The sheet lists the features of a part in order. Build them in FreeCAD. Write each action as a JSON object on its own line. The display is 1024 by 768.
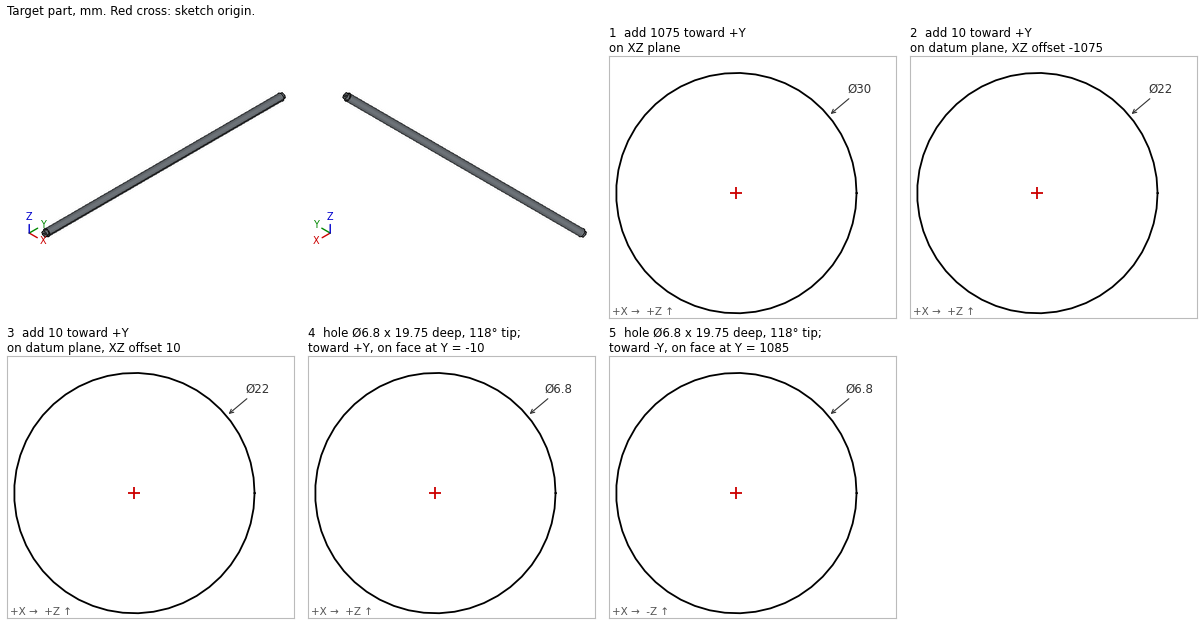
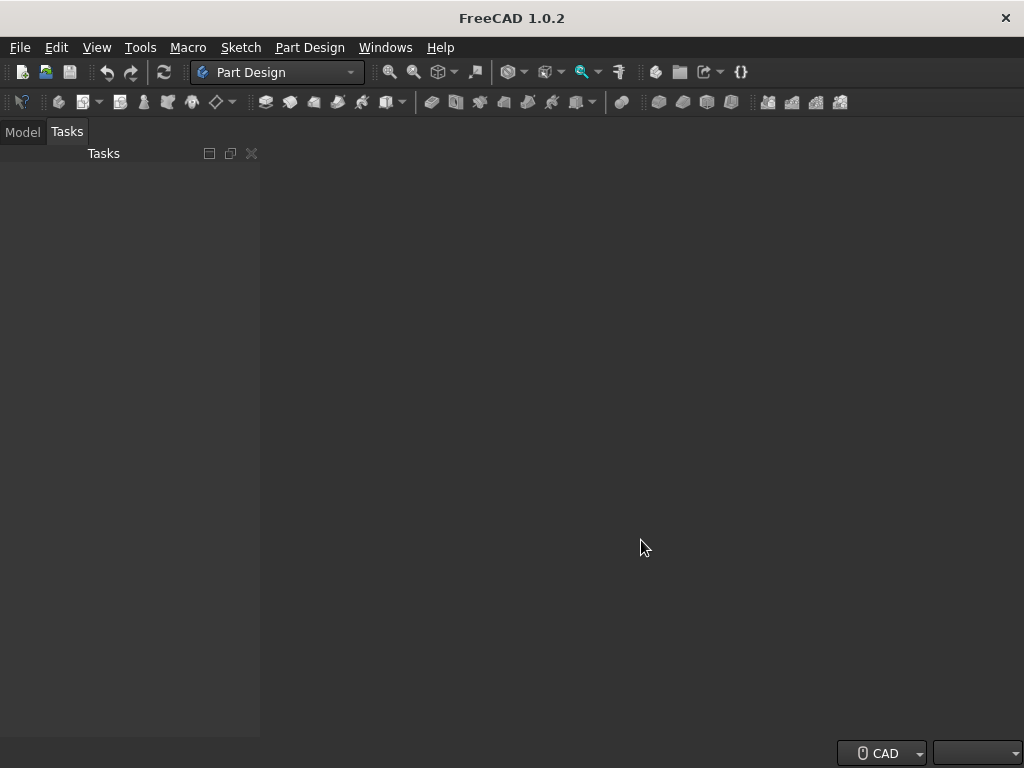
{"action": "left_click", "coordinate": [22, 72]}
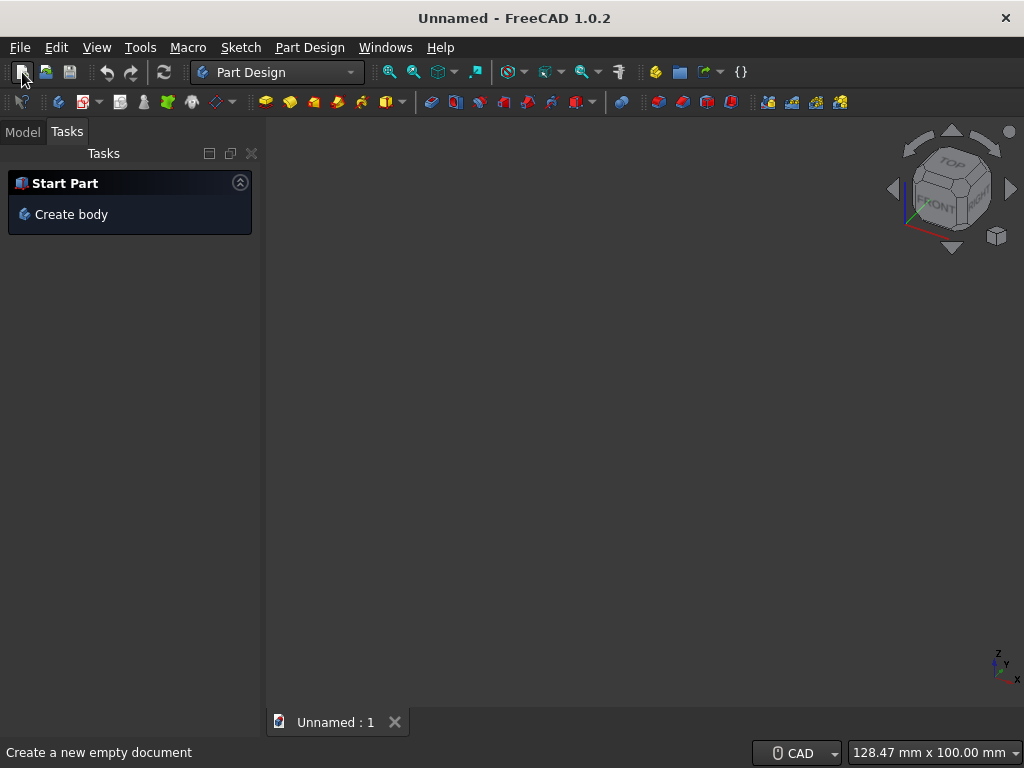
{"action": "left_click", "coordinate": [84, 102]}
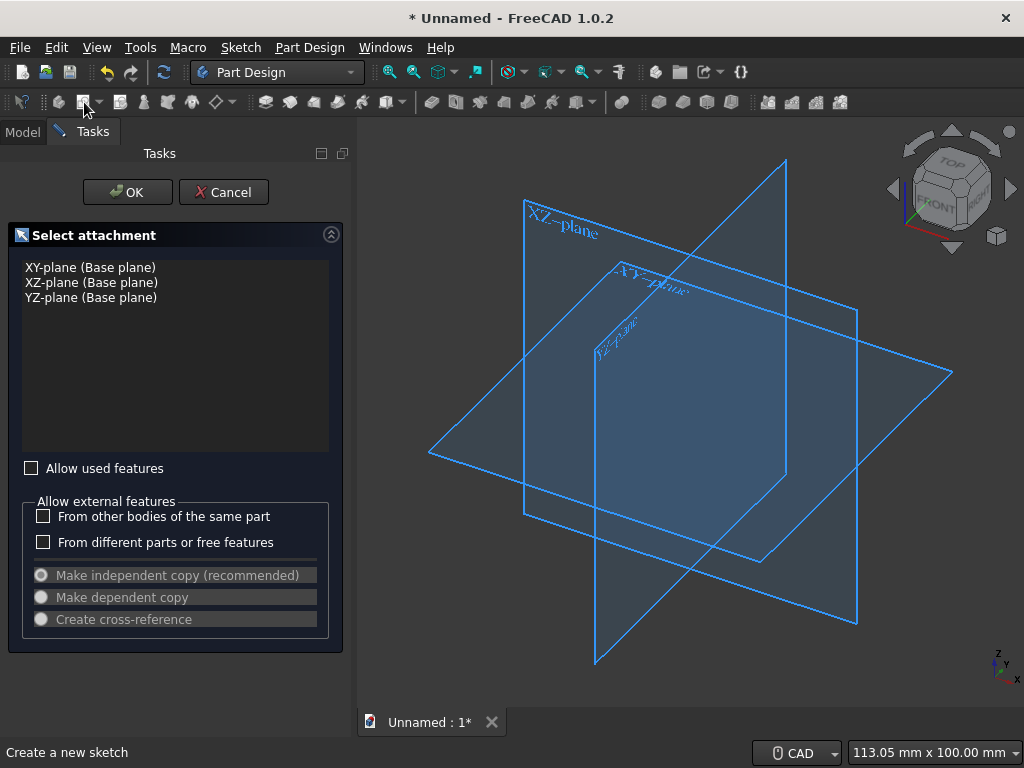
{"action": "left_click", "coordinate": [82, 282]}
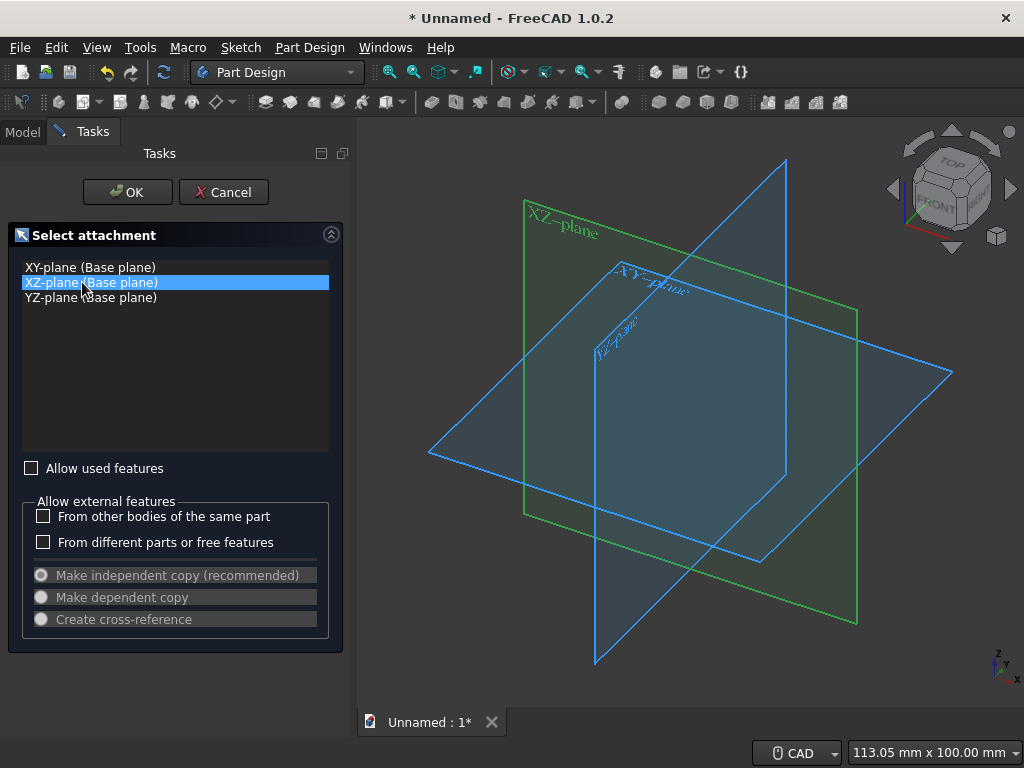
{"action": "left_click", "coordinate": [128, 192]}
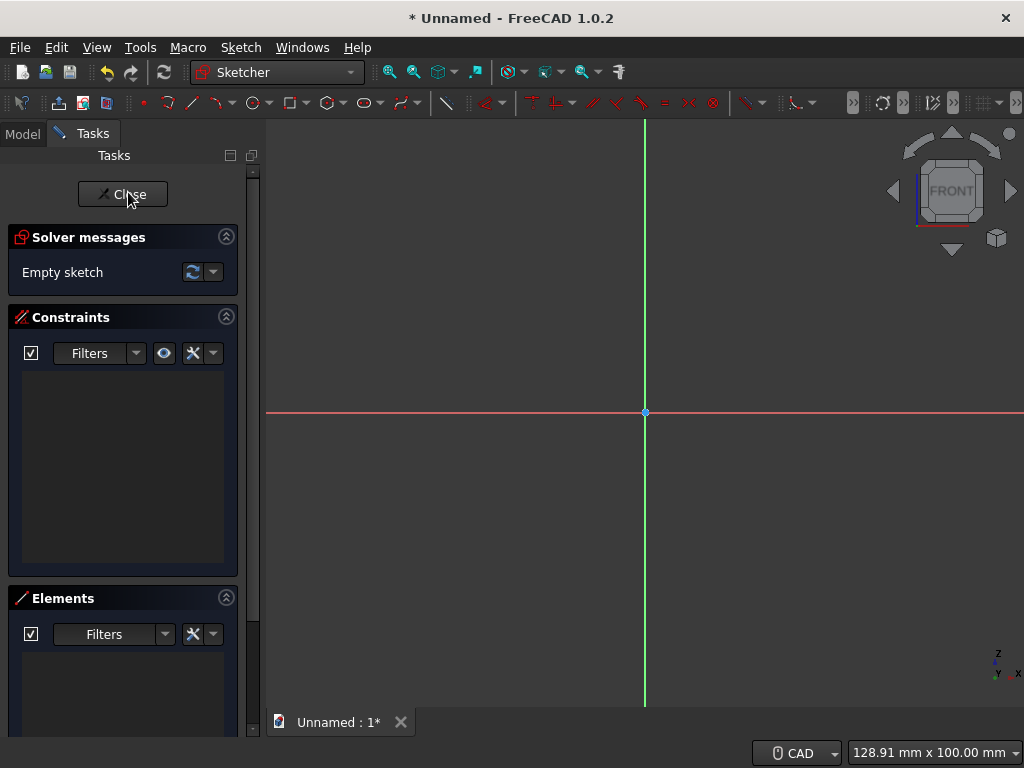
{"action": "scroll", "coordinate": [701, 413], "scroll_direction": "up", "scroll_amount": 4}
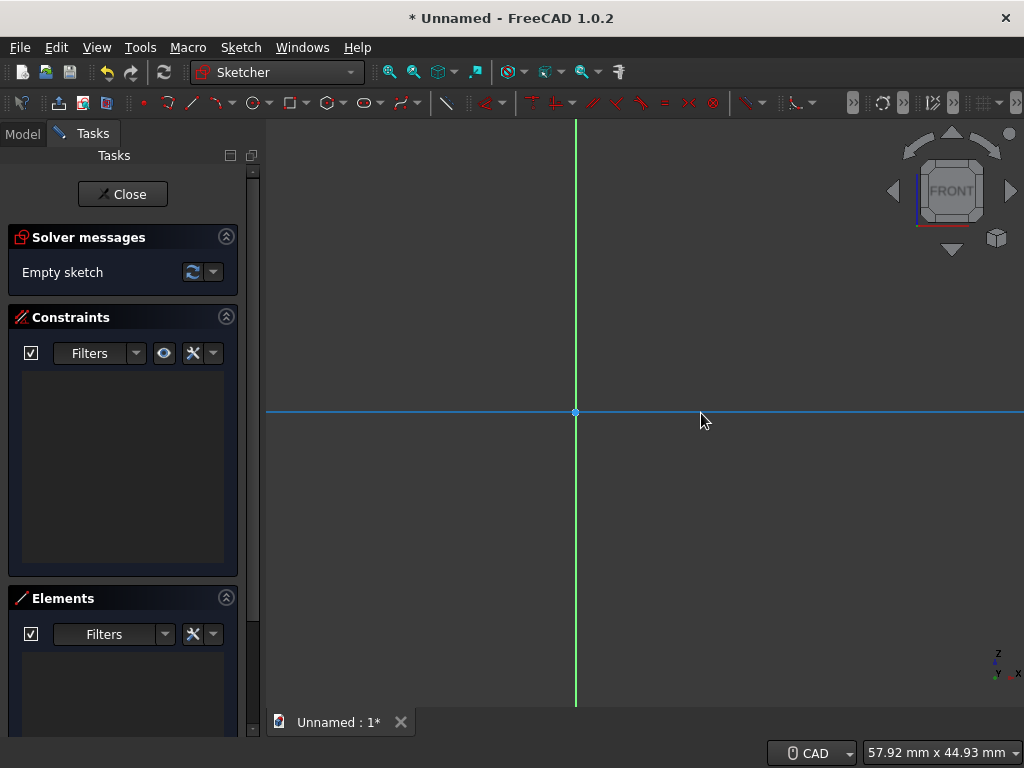
{"action": "left_click", "coordinate": [254, 104]}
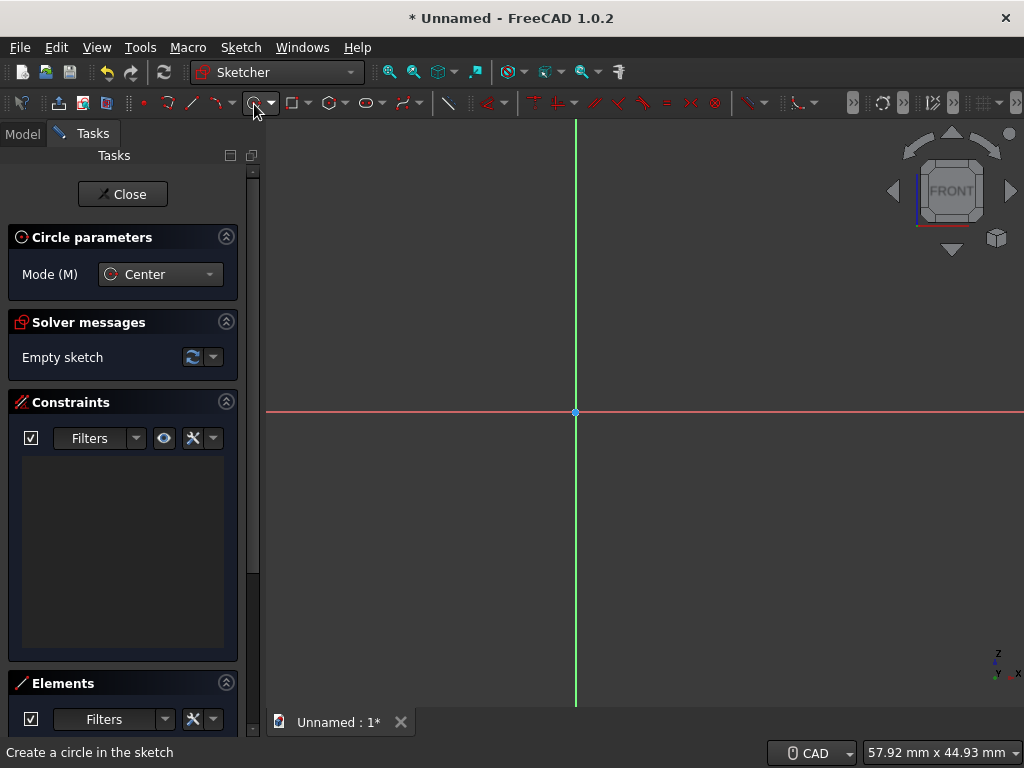
{"action": "left_click", "coordinate": [576, 412]}
{"action": "mouse_move", "coordinate": [714, 274]}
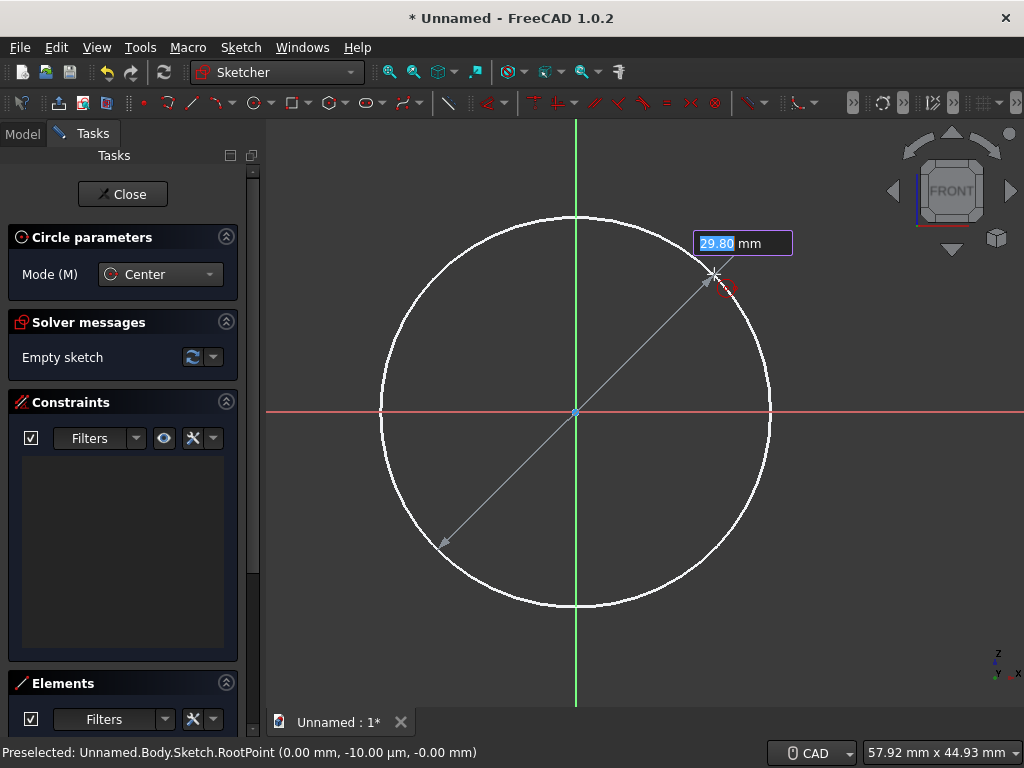
{"action": "type", "text": "30"}
{"action": "key", "text": "Return"}
{"action": "key", "text": "Escape"}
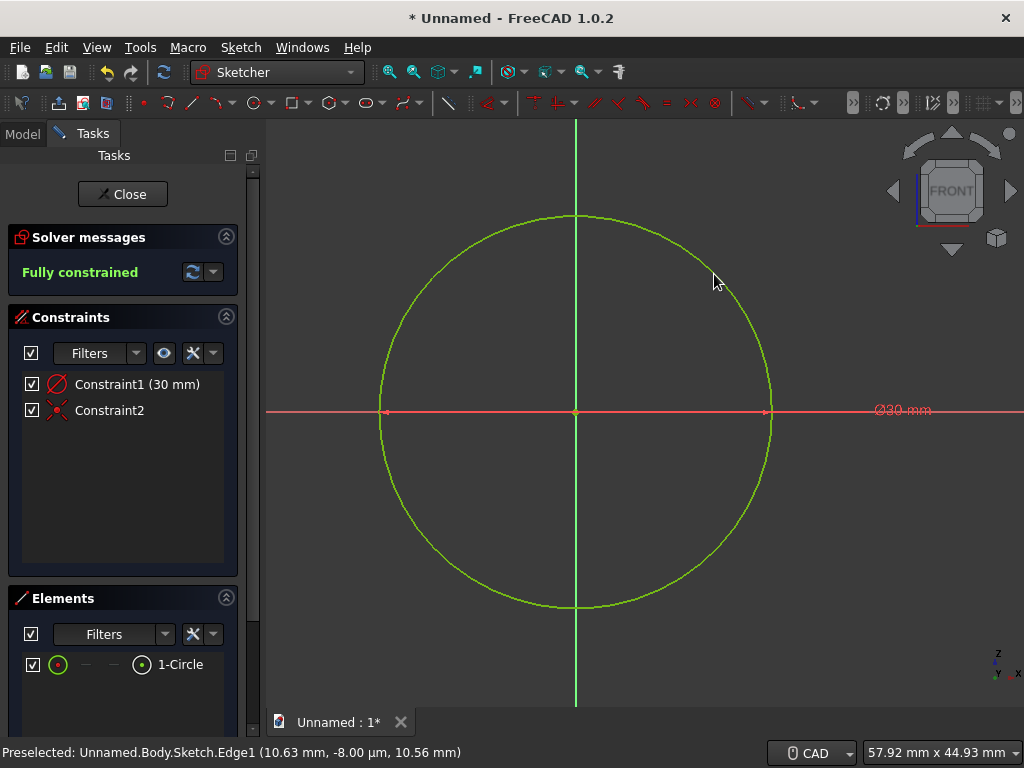
{"action": "left_click", "coordinate": [123, 194]}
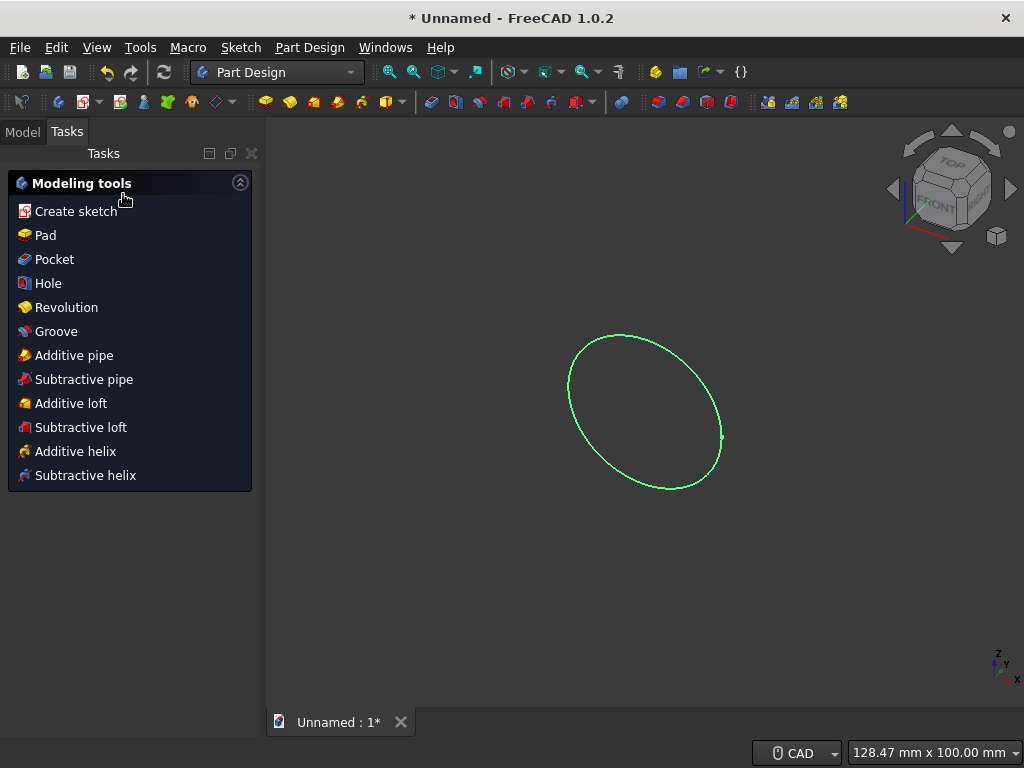
{"action": "left_click", "coordinate": [266, 102]}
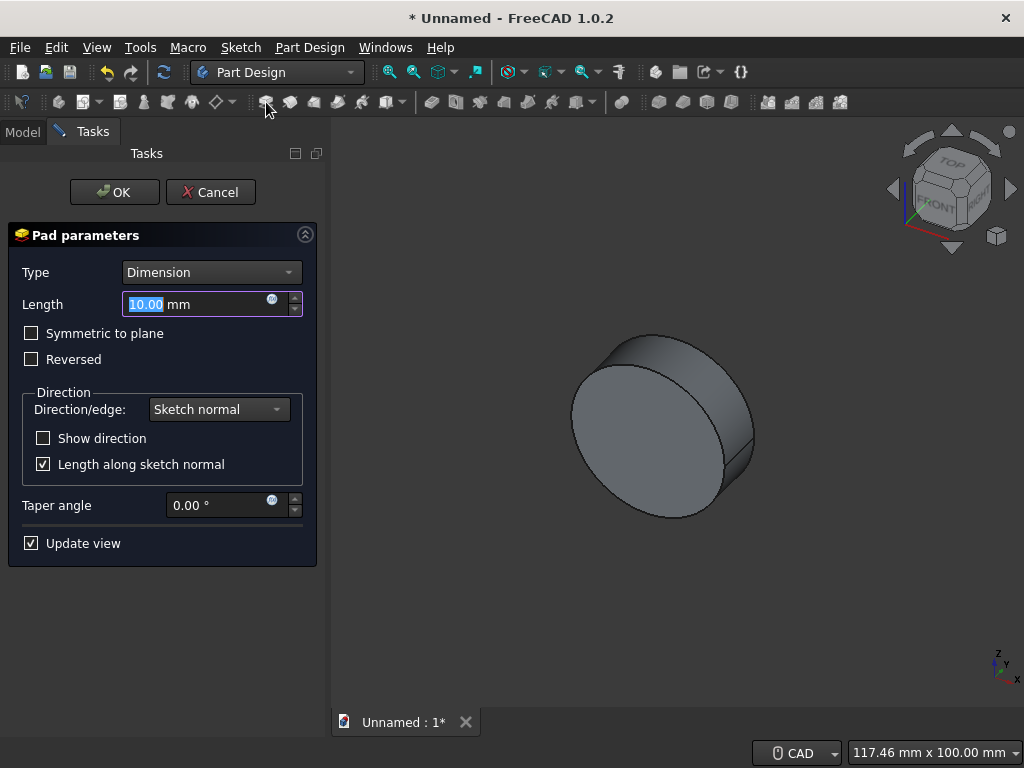
{"action": "type", "text": "1075"}
{"action": "key", "text": "Tab"}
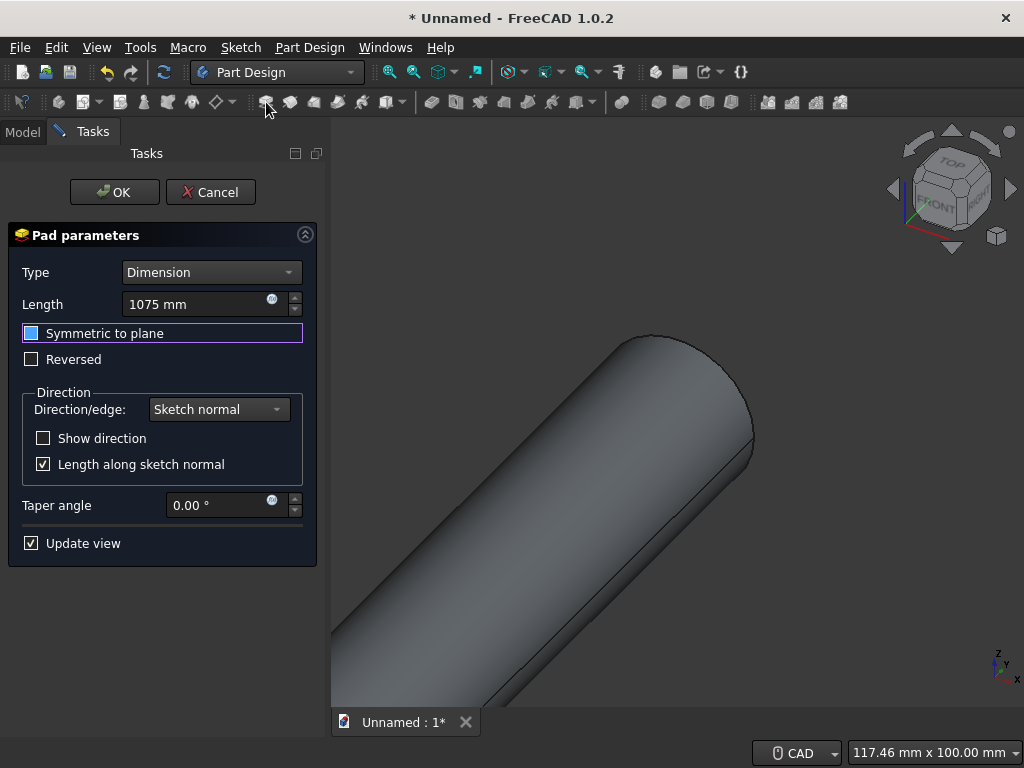
{"action": "left_click", "coordinate": [30, 359]}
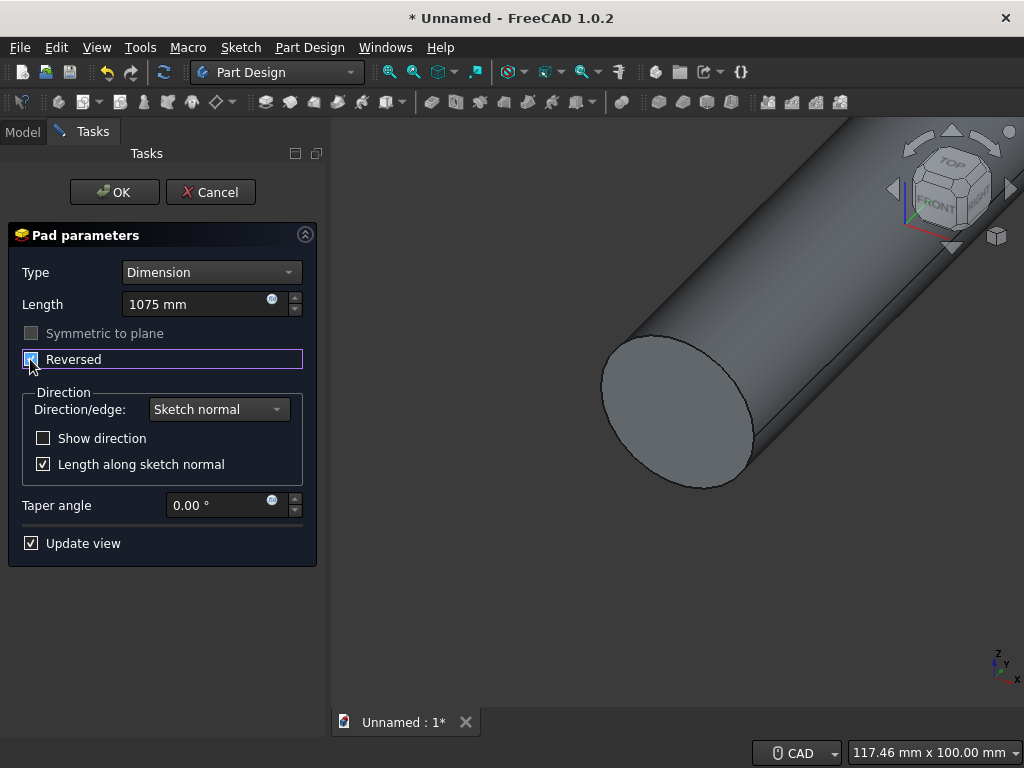
{"action": "left_click", "coordinate": [115, 192]}